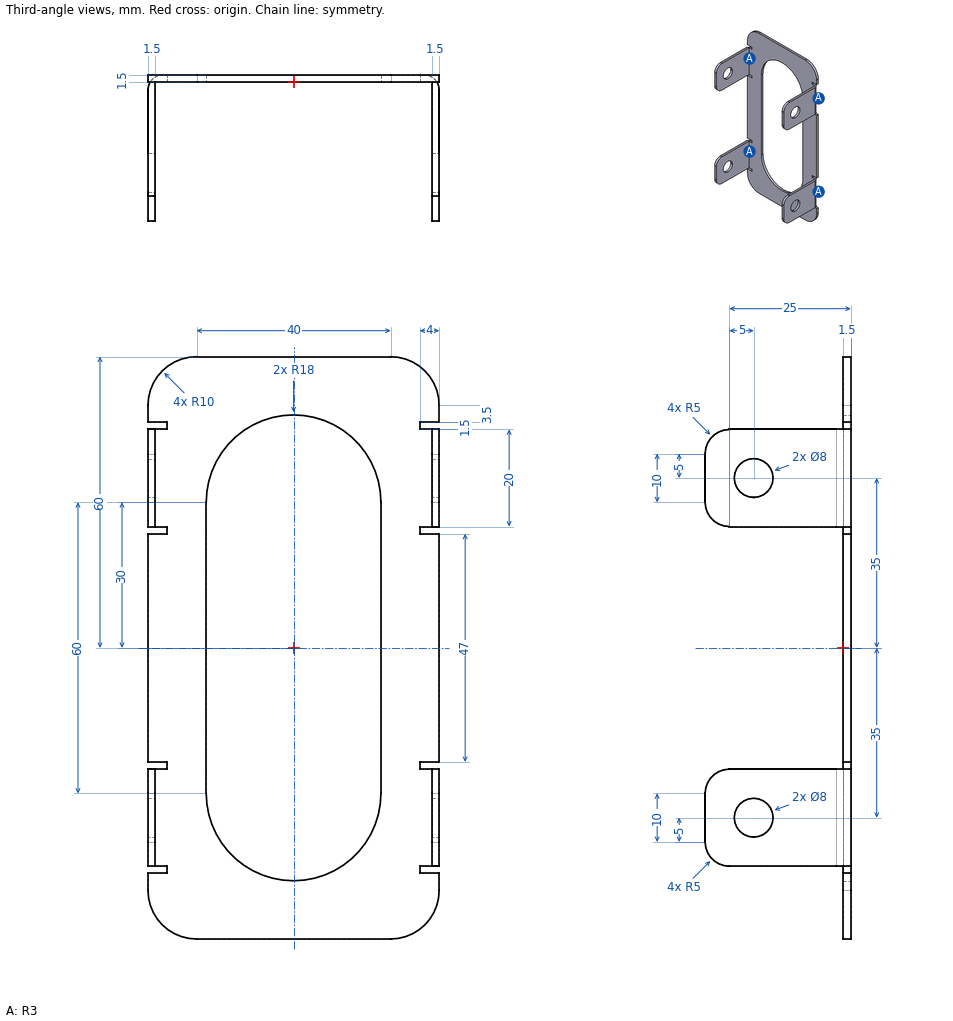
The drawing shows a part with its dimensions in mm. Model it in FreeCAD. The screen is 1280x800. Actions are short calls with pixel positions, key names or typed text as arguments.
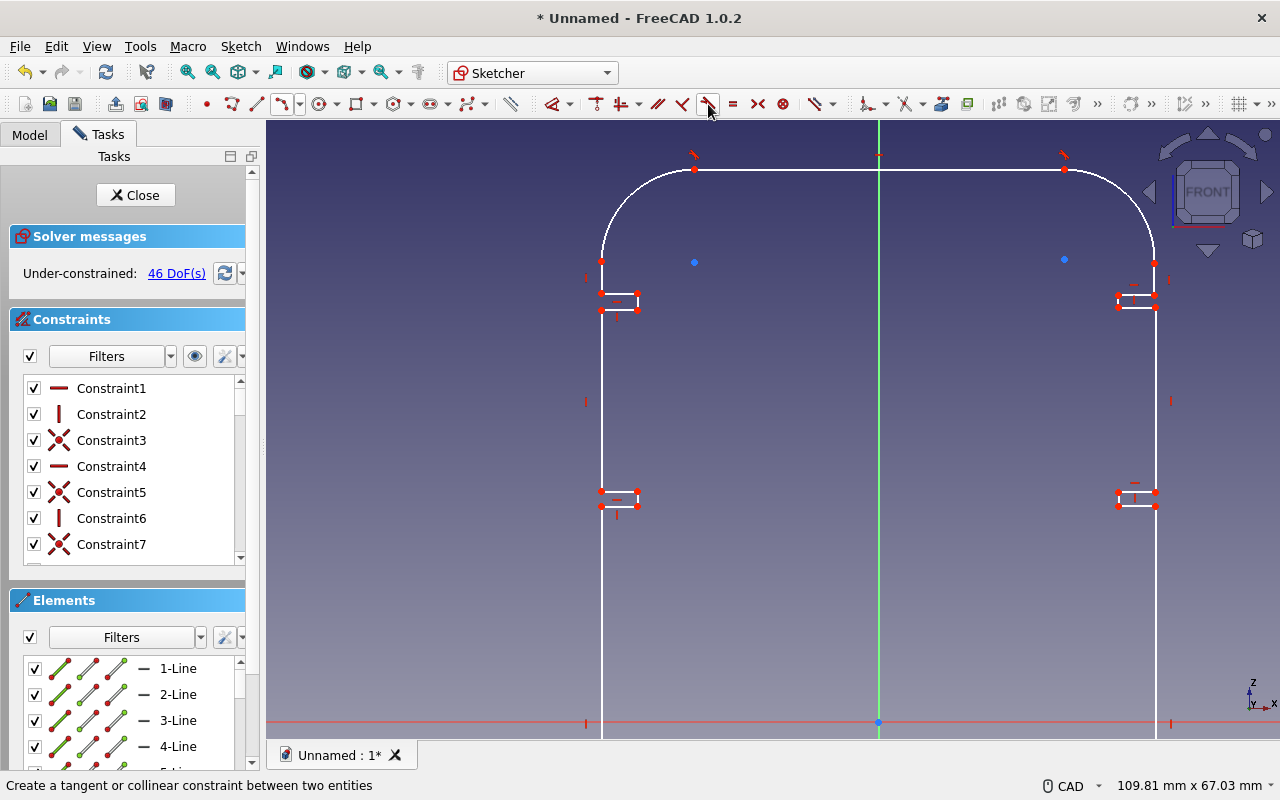
scroll(603, 259, down, 5)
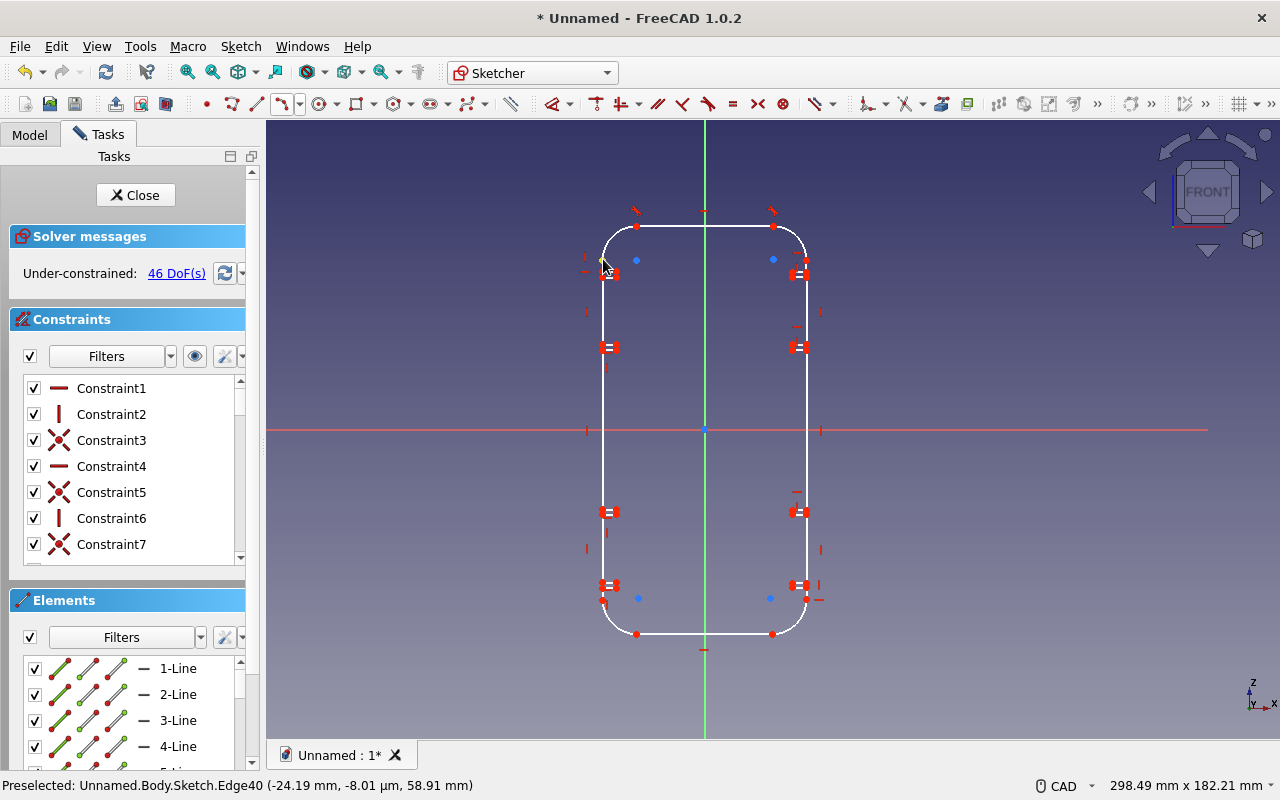
scroll(806, 264, up, 7)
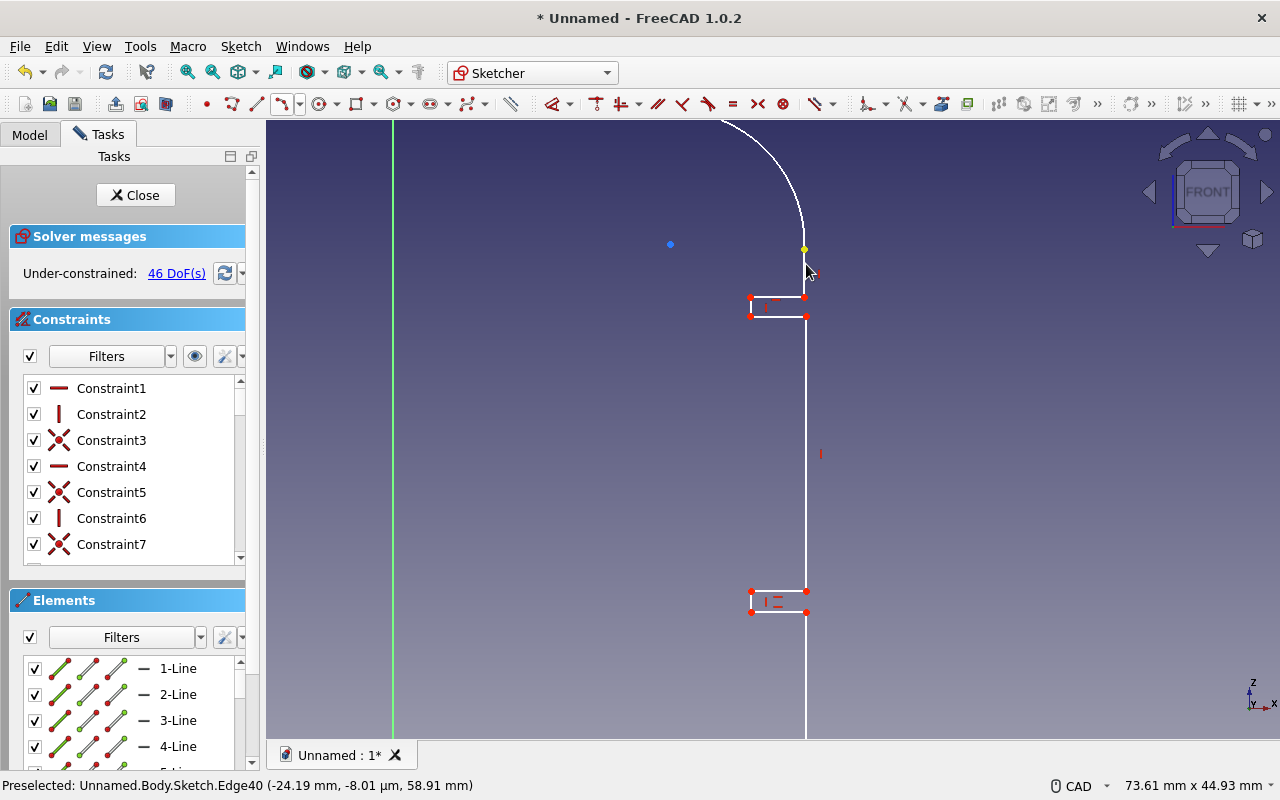
click(804, 264)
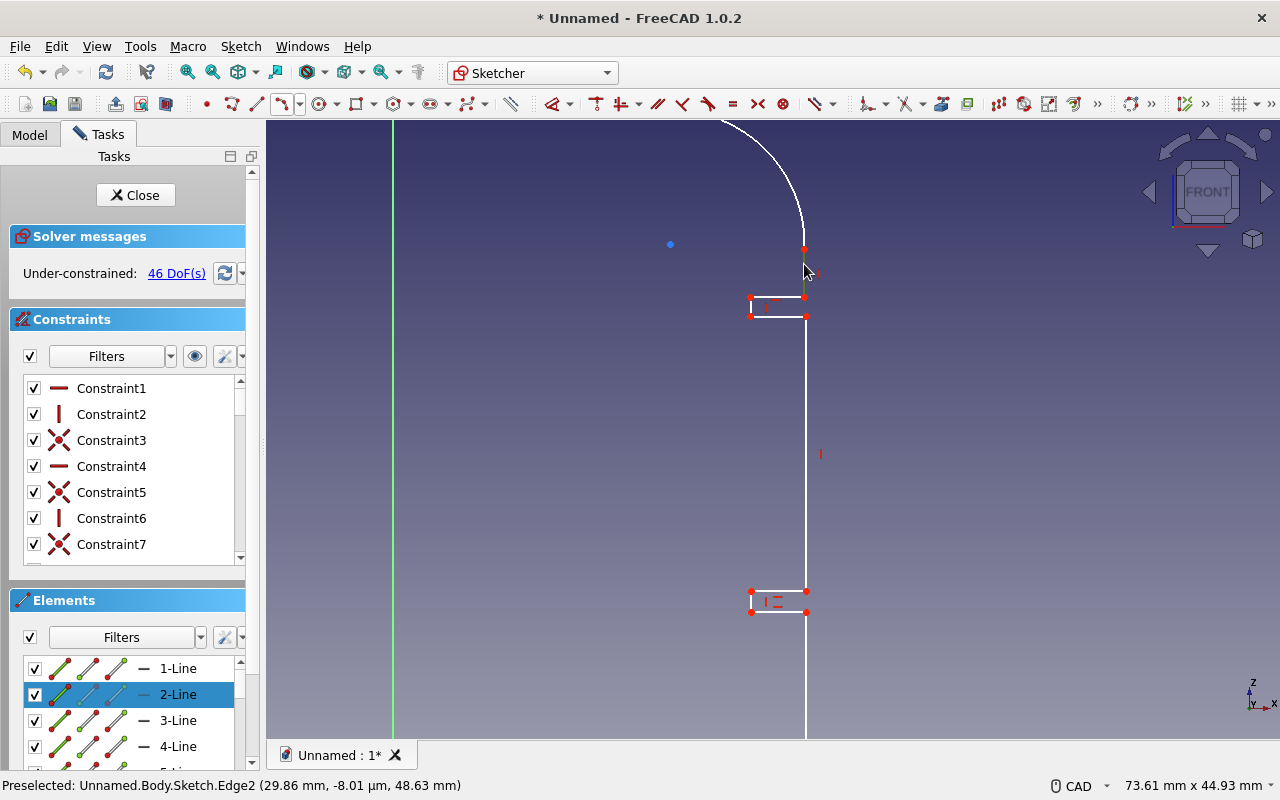
scroll(806, 264, down, 7)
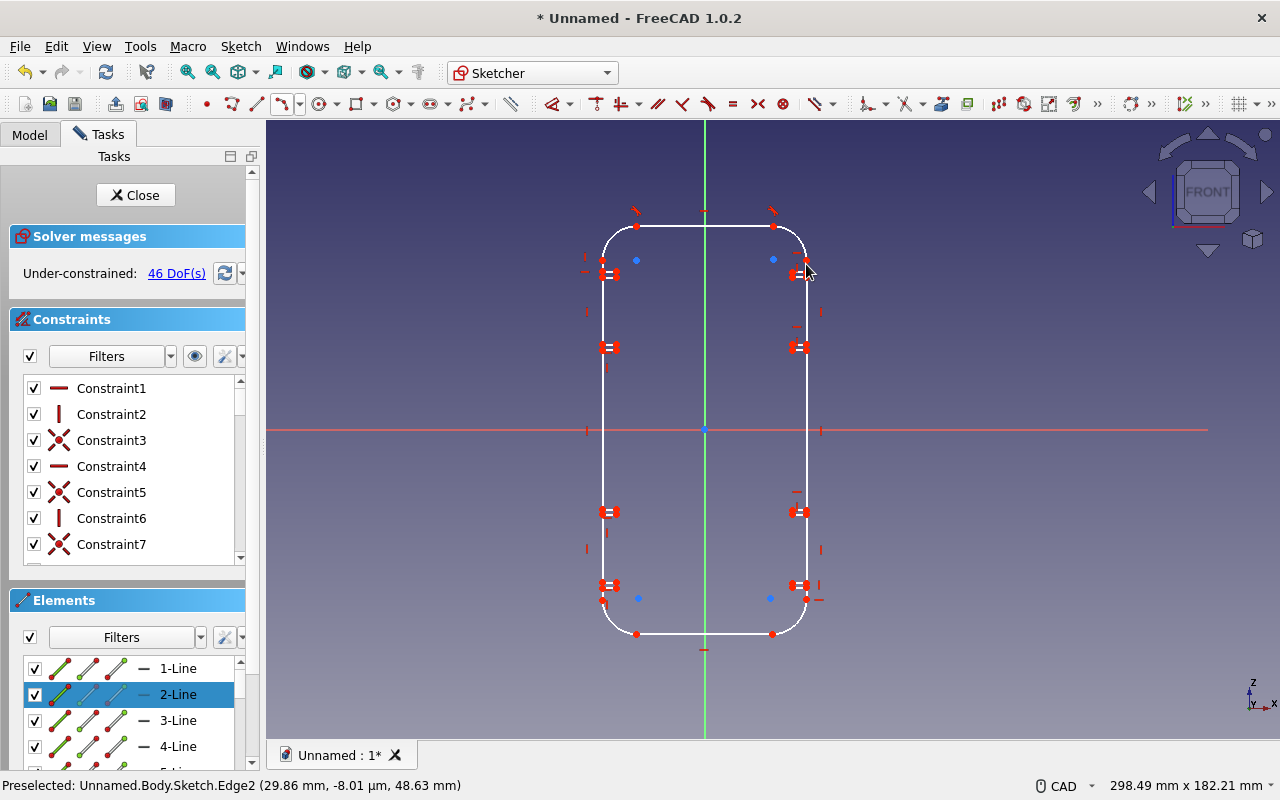
click(803, 245)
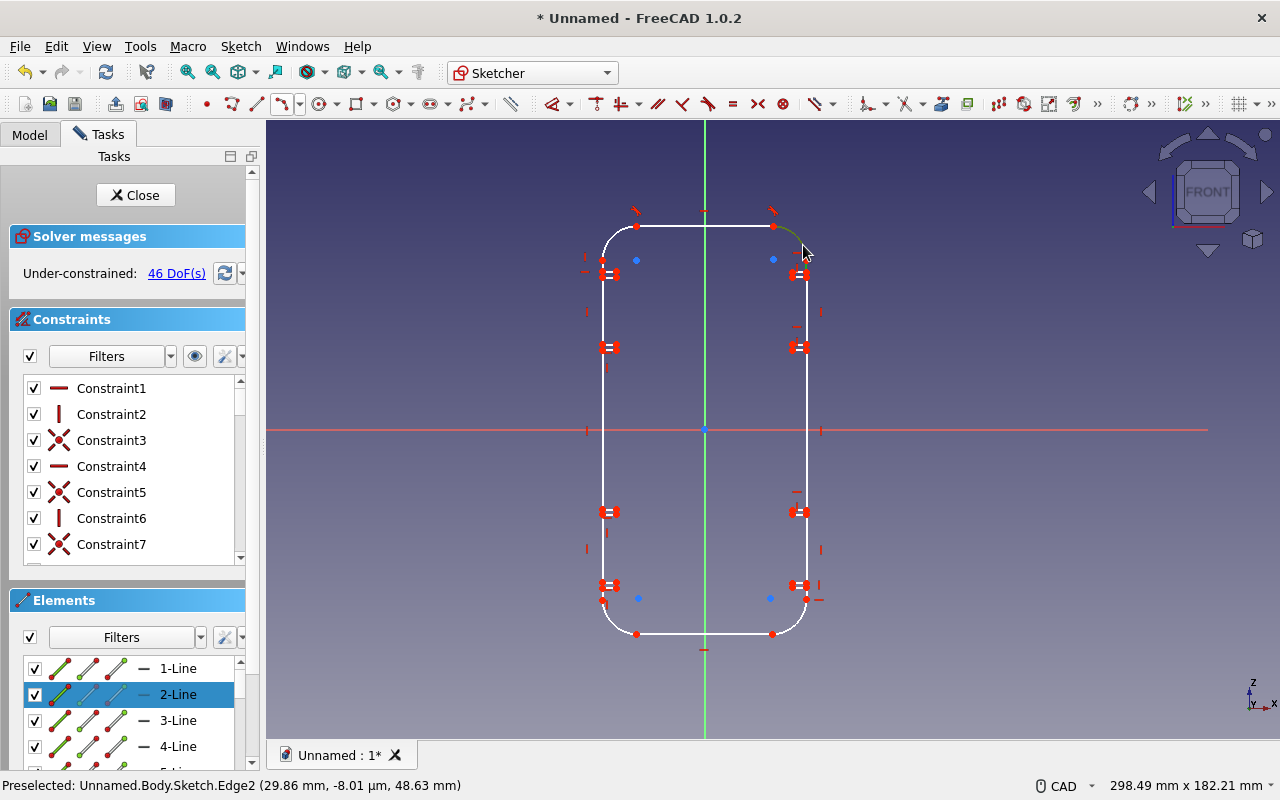
click(708, 104)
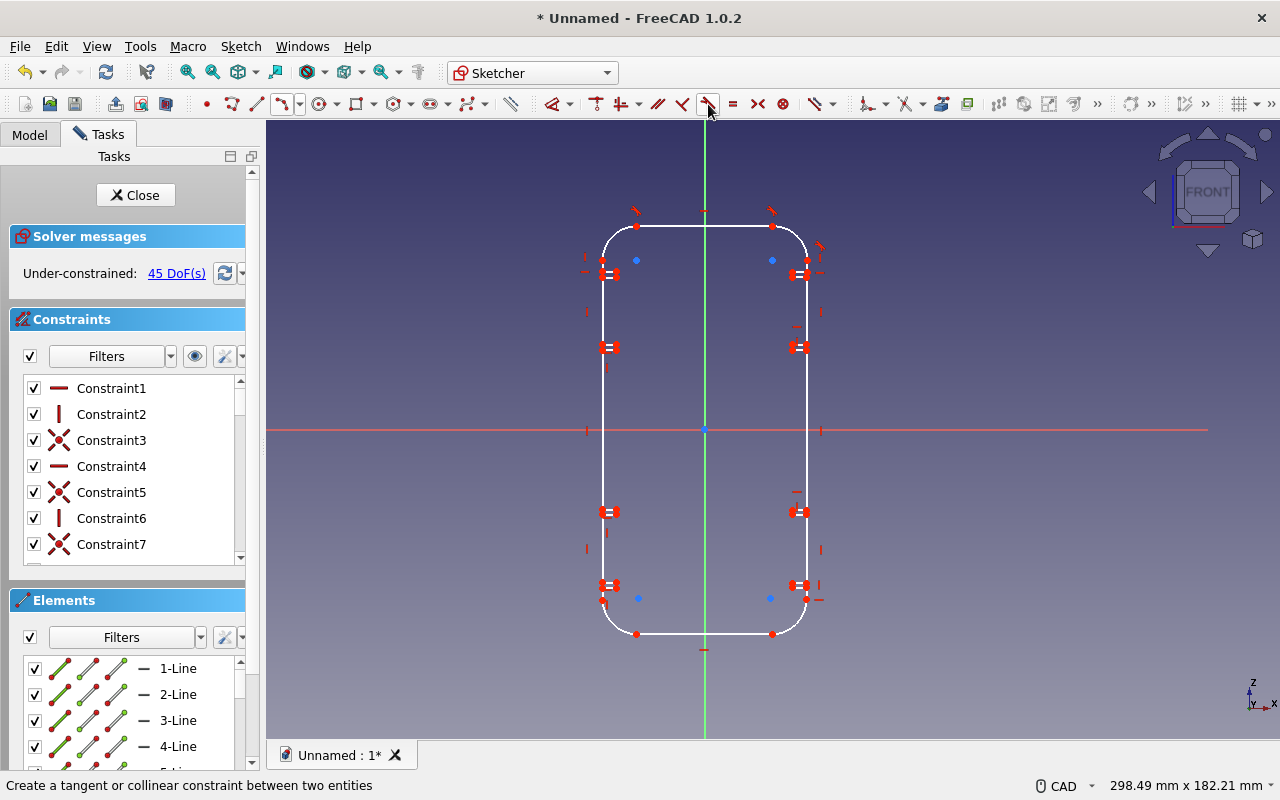
scroll(807, 594, up, 5)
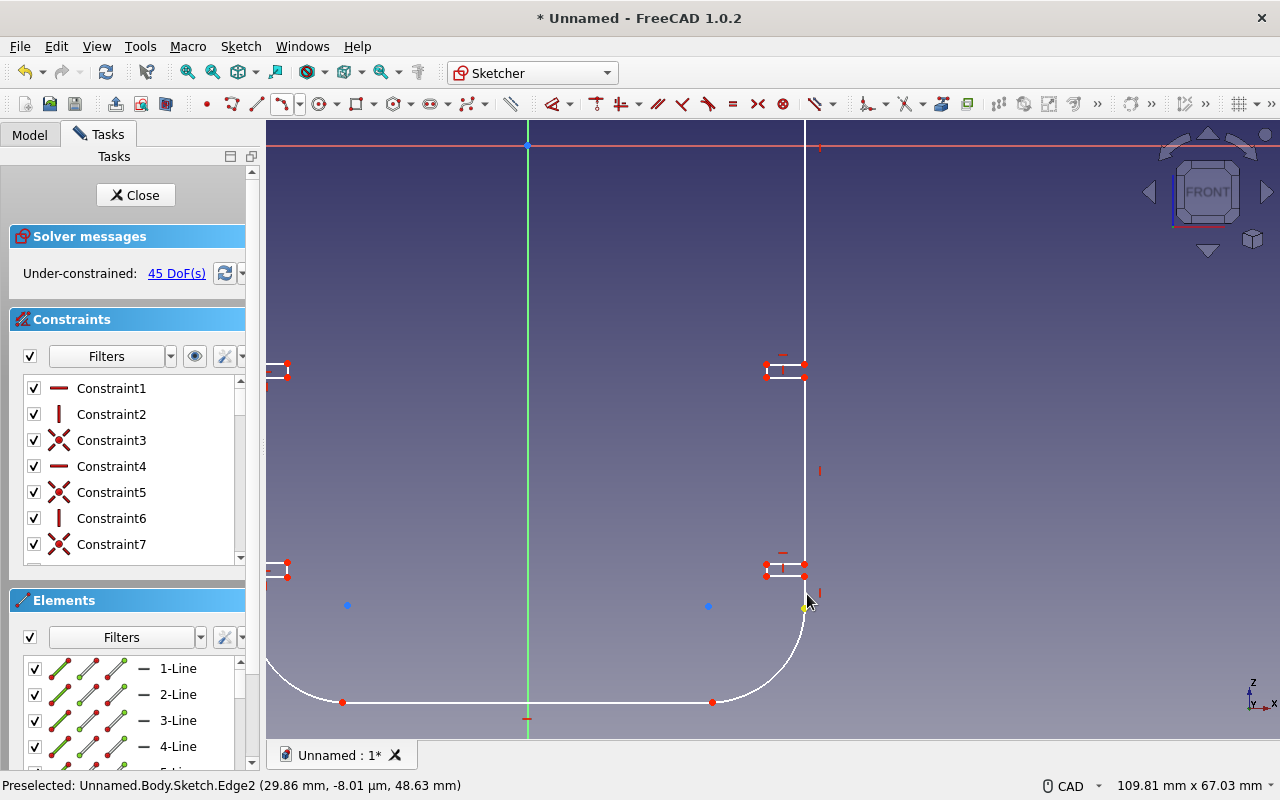
click(805, 592)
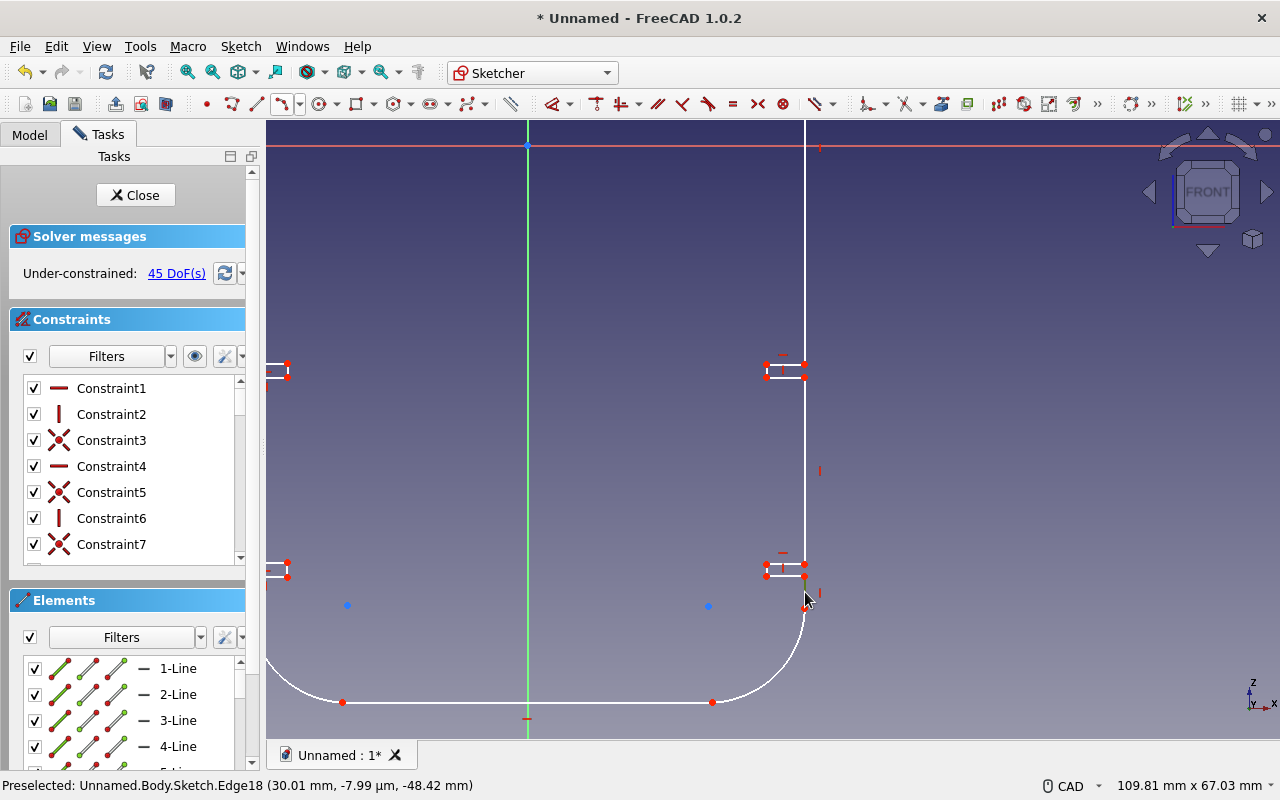
click(754, 691)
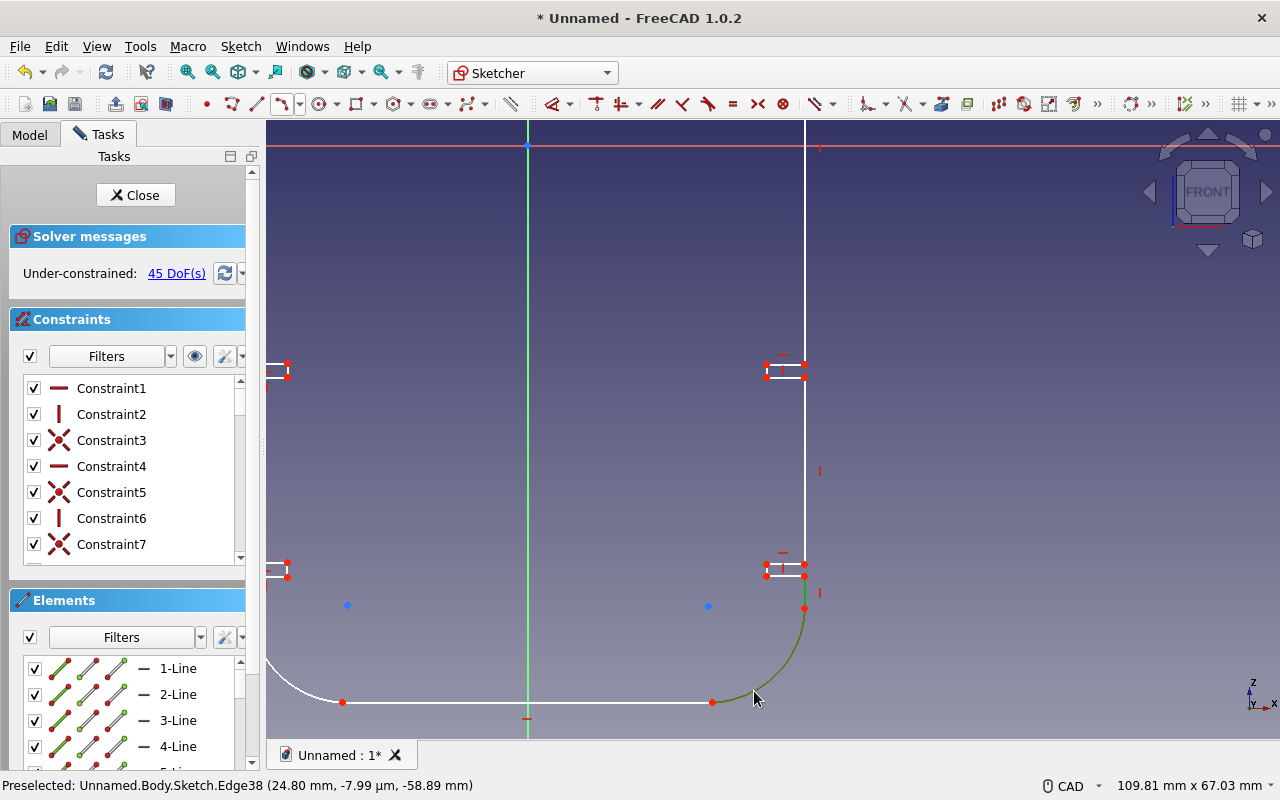
click(708, 104)